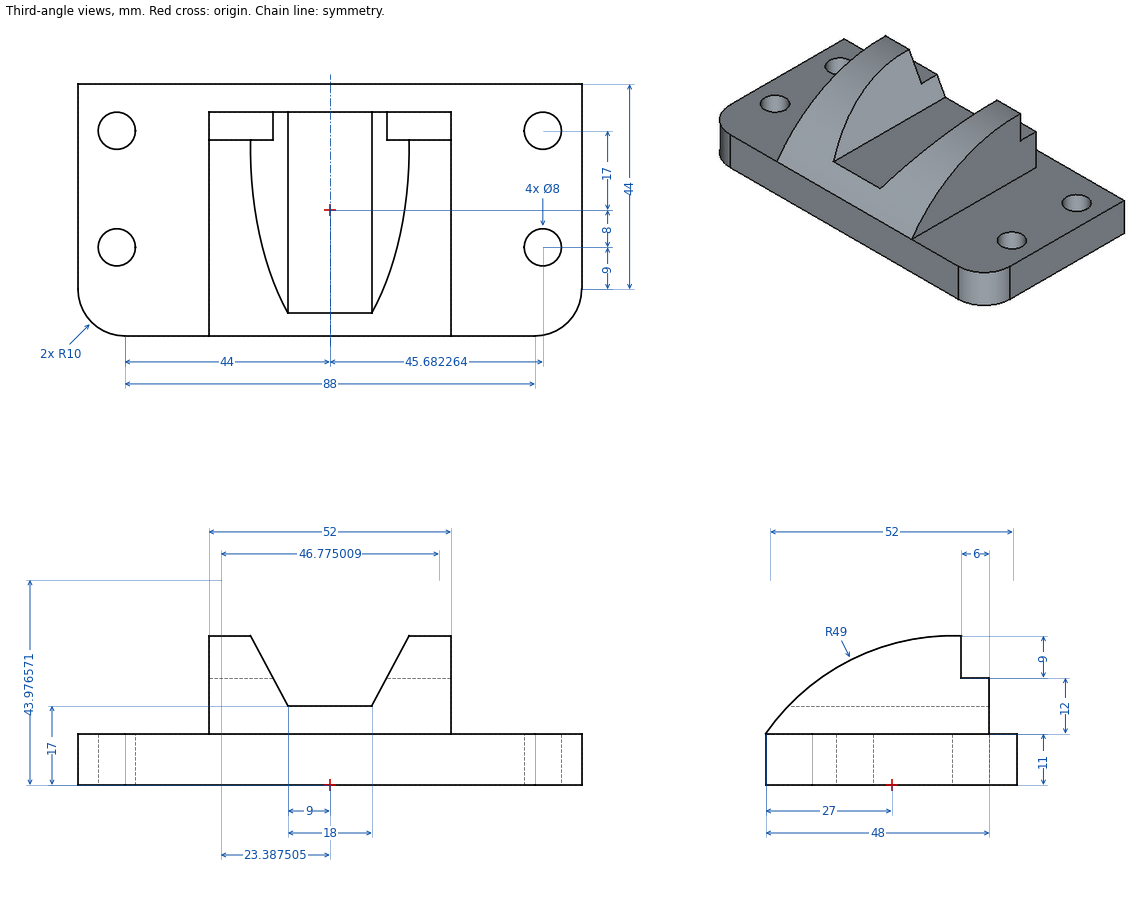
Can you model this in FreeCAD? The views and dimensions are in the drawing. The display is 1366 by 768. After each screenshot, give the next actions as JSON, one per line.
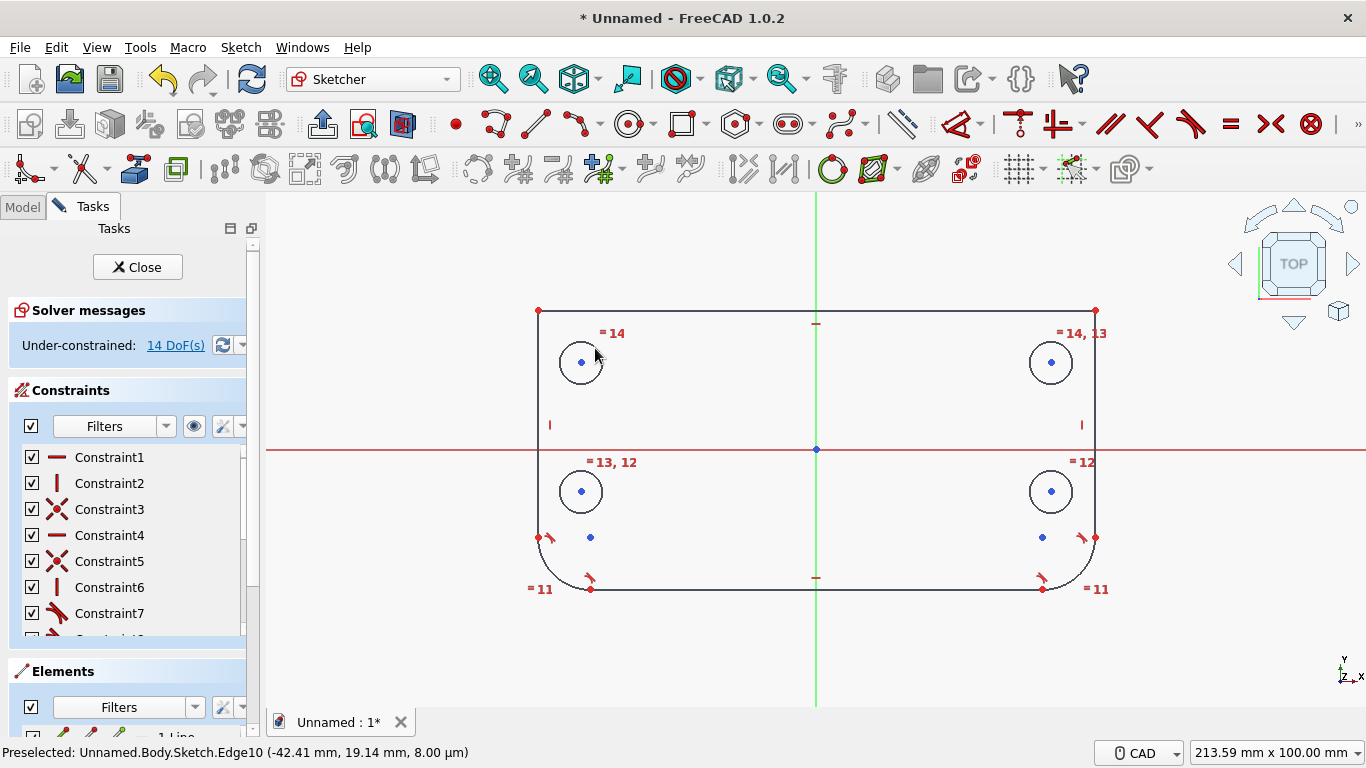
{"action": "left_click", "coordinate": [1051, 492]}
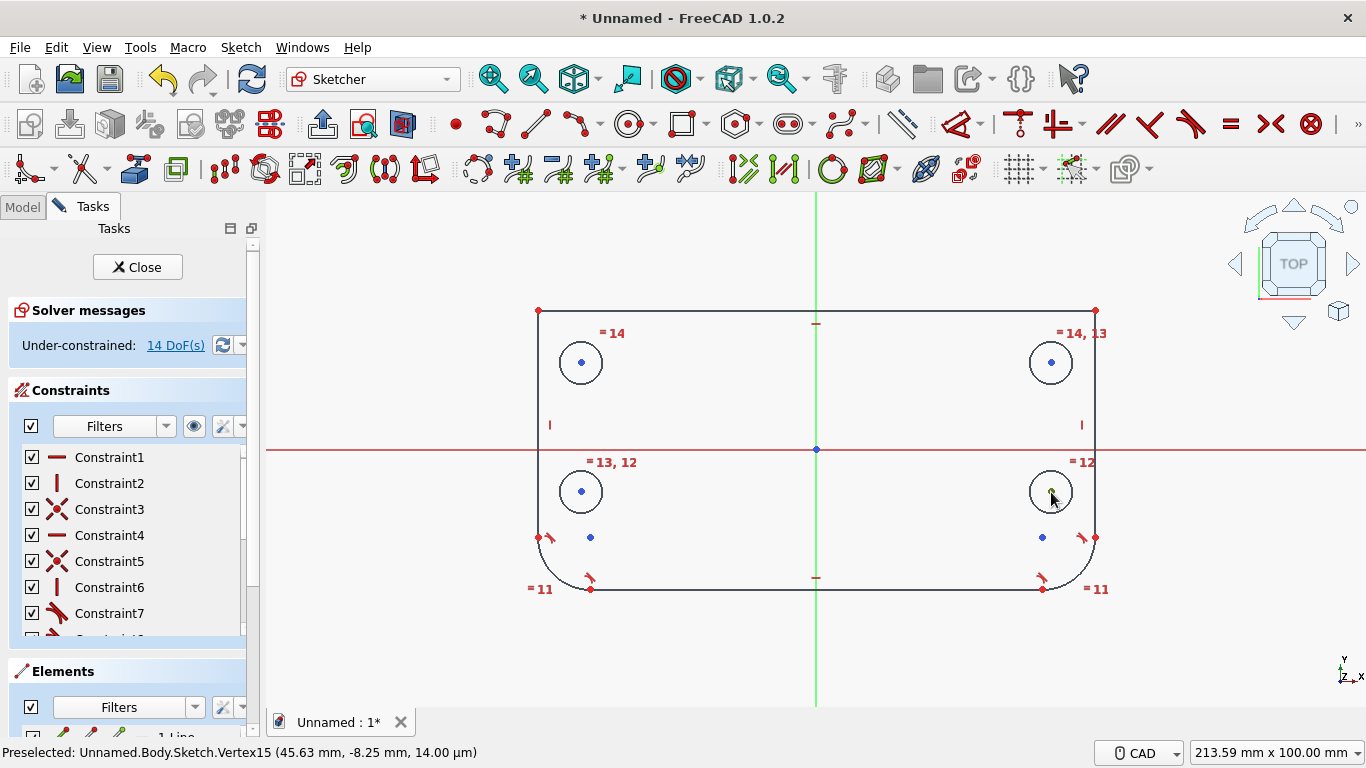
{"action": "left_click", "coordinate": [581, 492]}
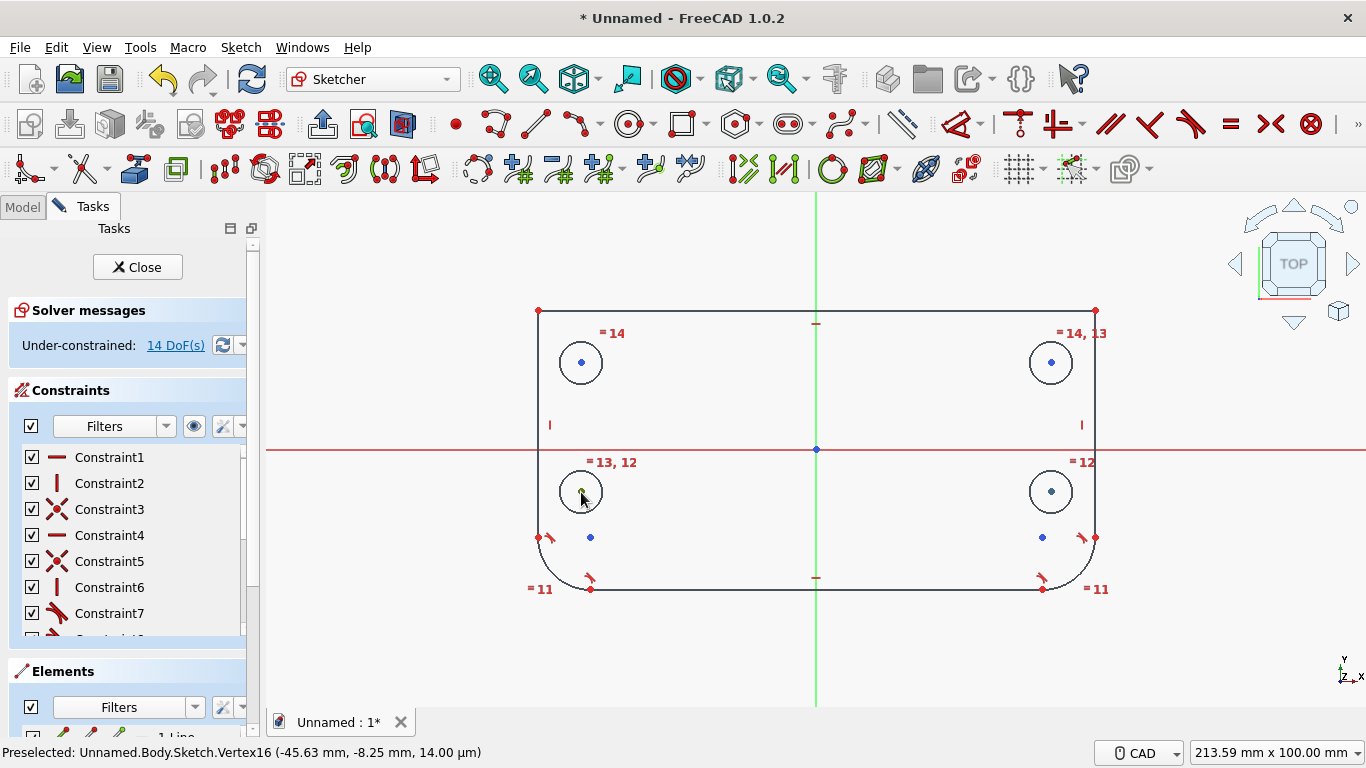
{"action": "left_click", "coordinate": [816, 646]}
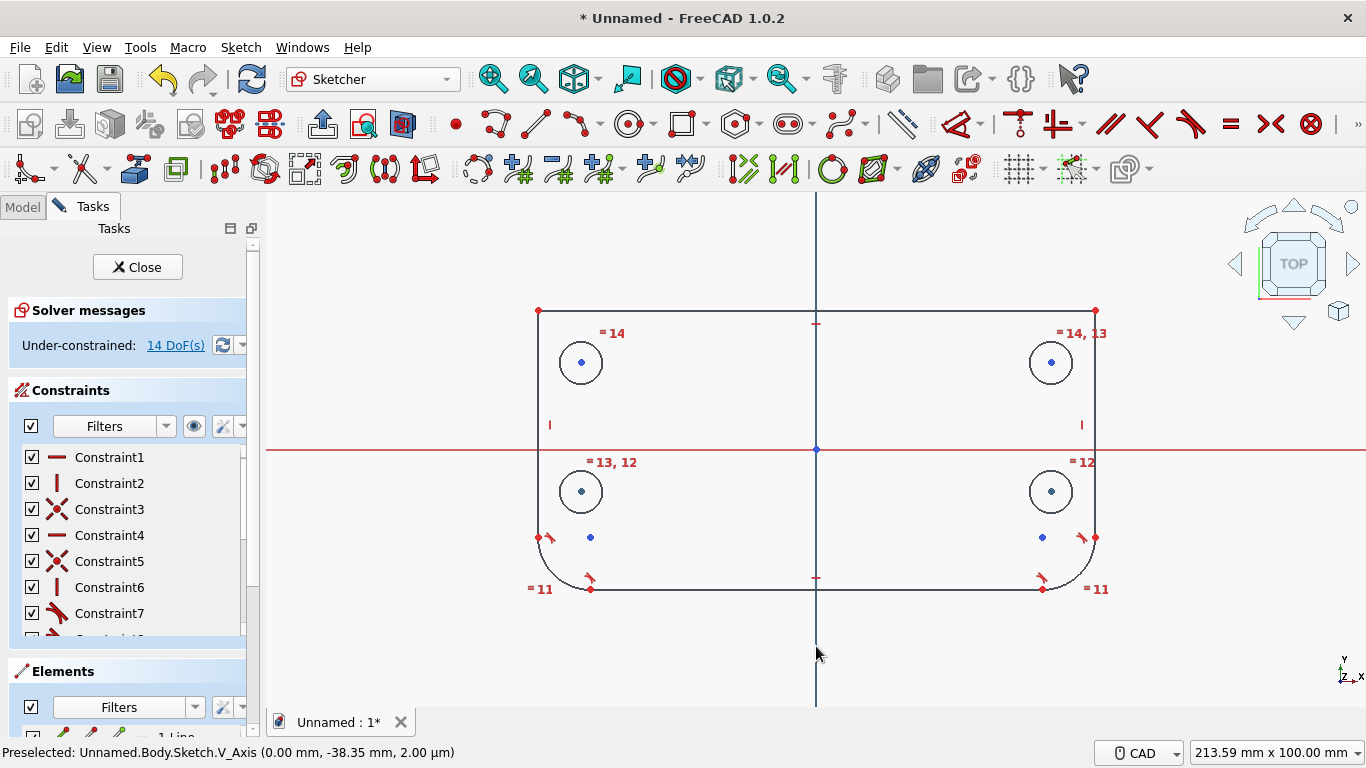
{"action": "left_click", "coordinate": [1272, 124]}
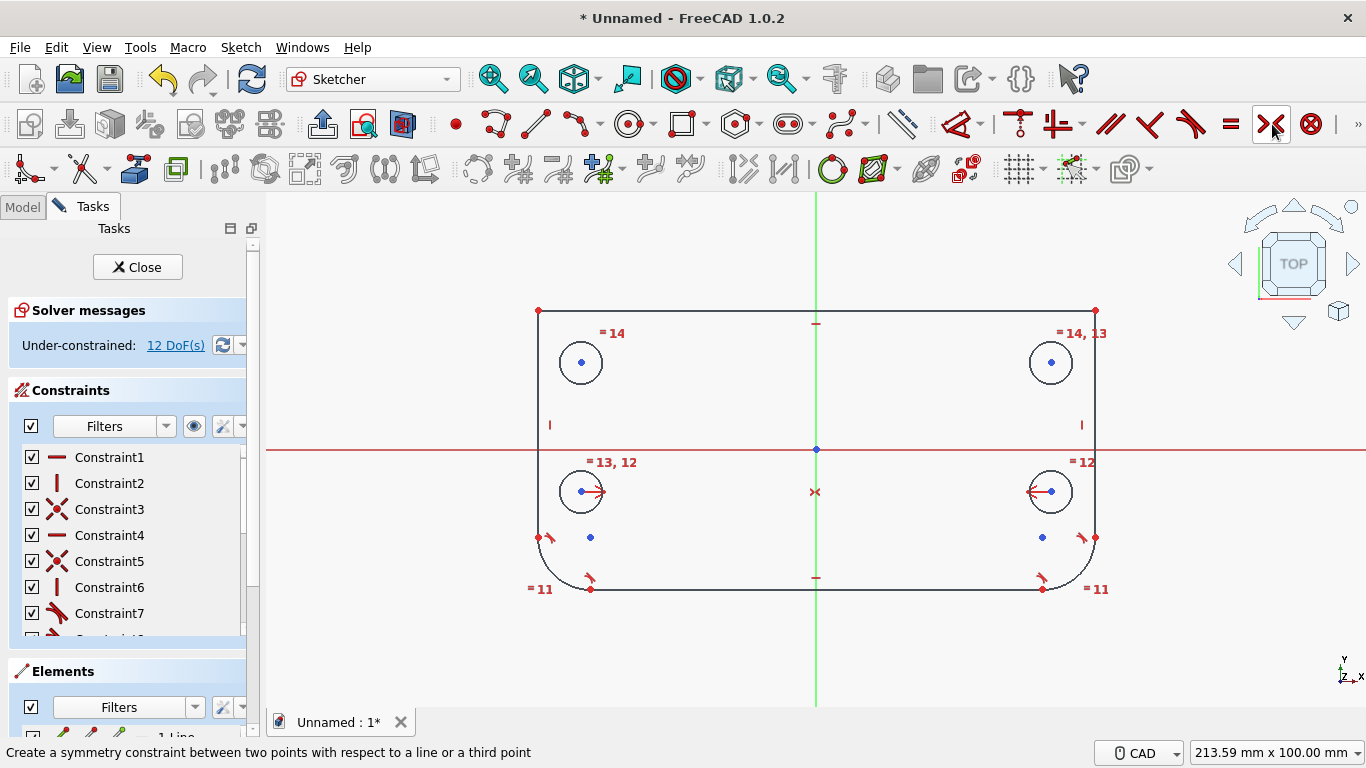
{"action": "left_click", "coordinate": [1051, 363]}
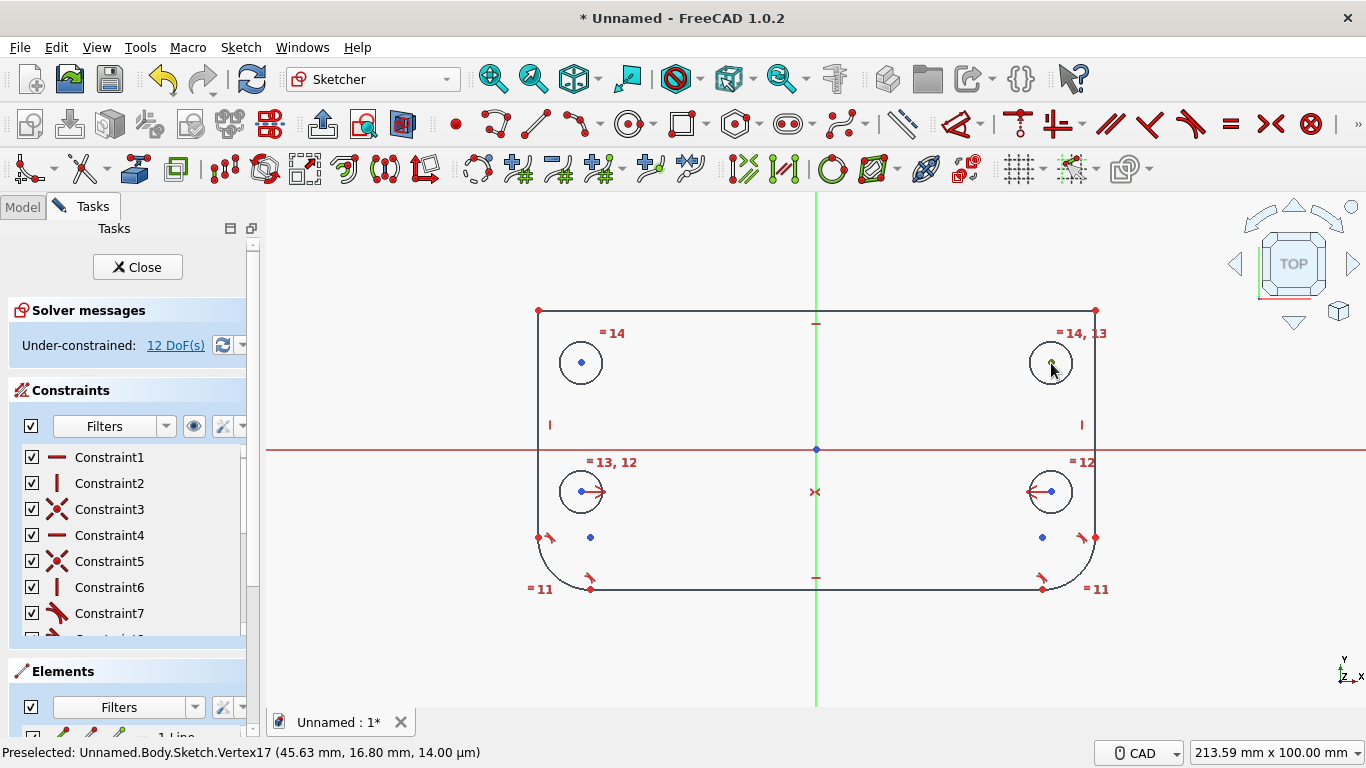
{"action": "left_click", "coordinate": [581, 363]}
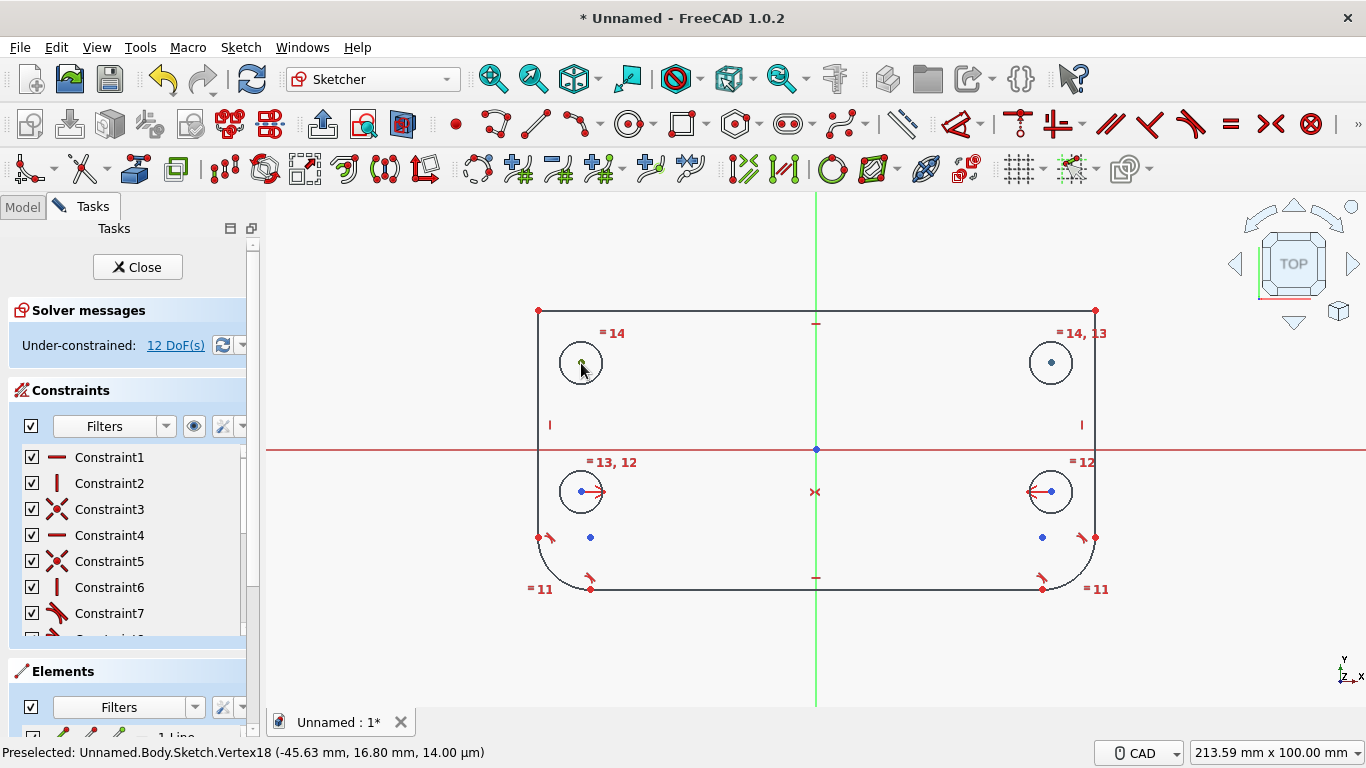
{"action": "left_click", "coordinate": [816, 646]}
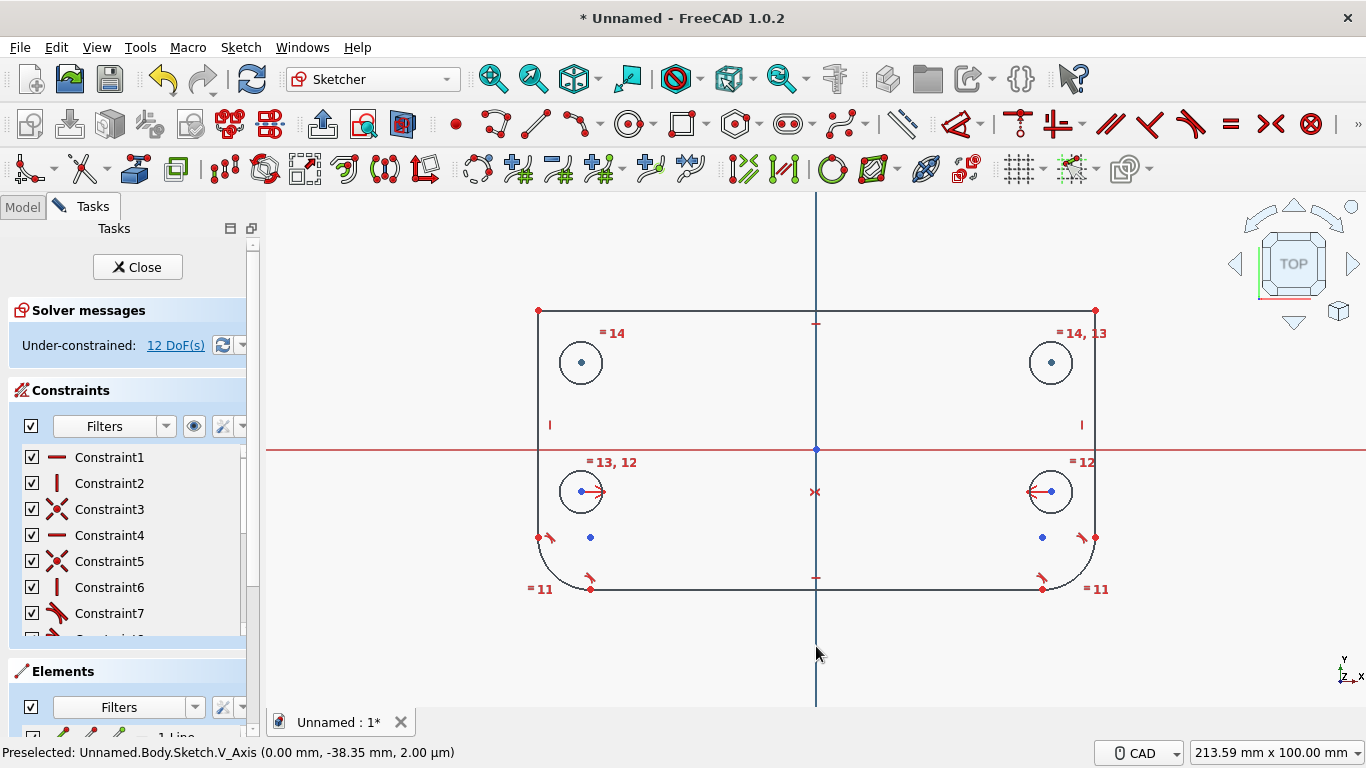
{"action": "key", "text": "s"}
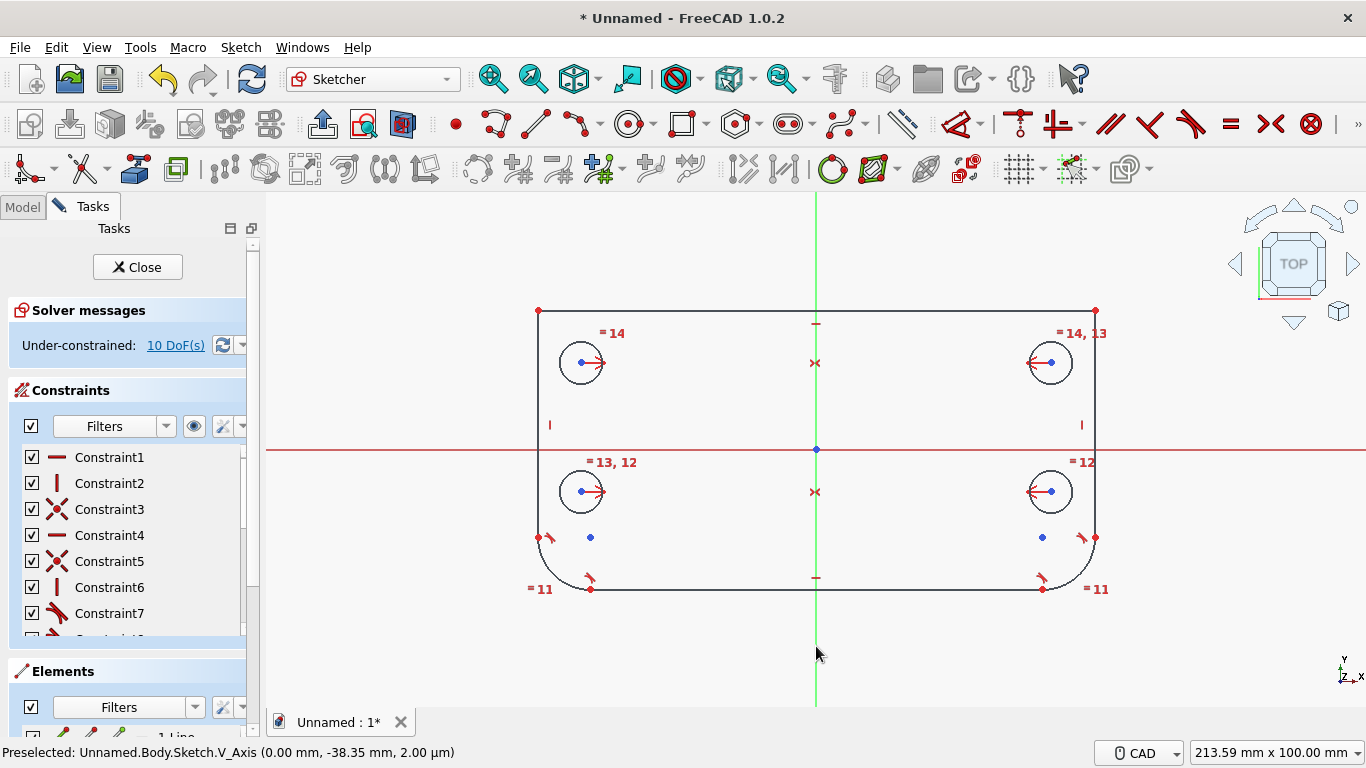
{"action": "key", "text": "d"}